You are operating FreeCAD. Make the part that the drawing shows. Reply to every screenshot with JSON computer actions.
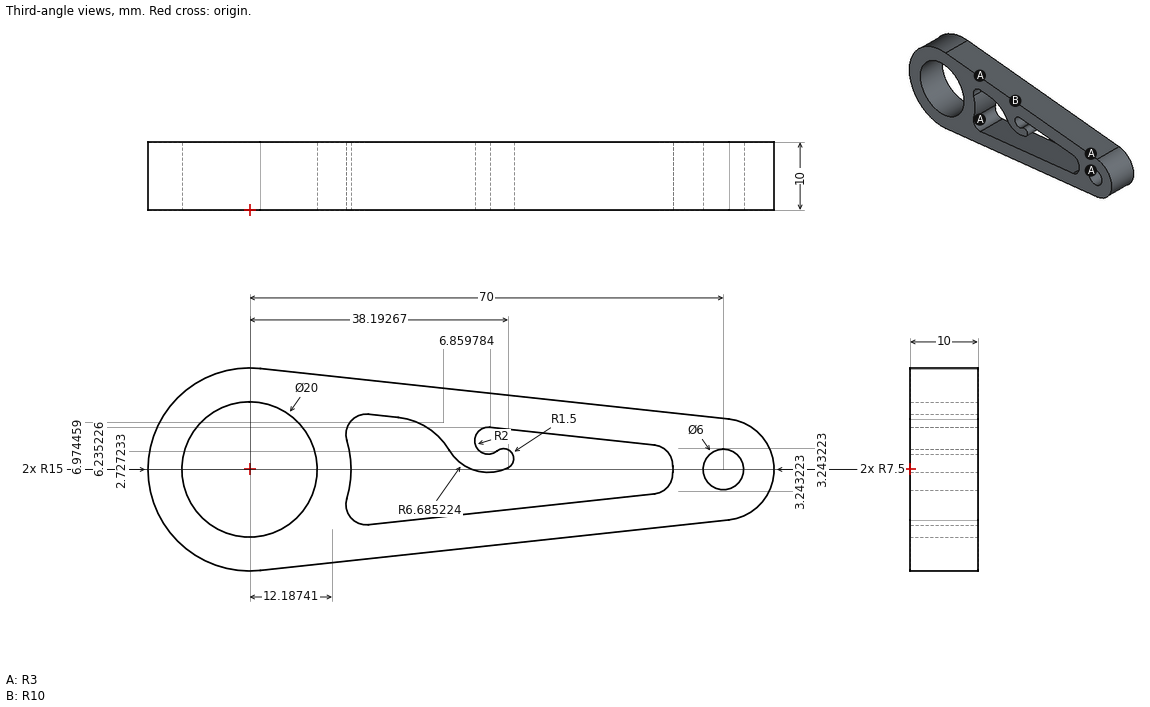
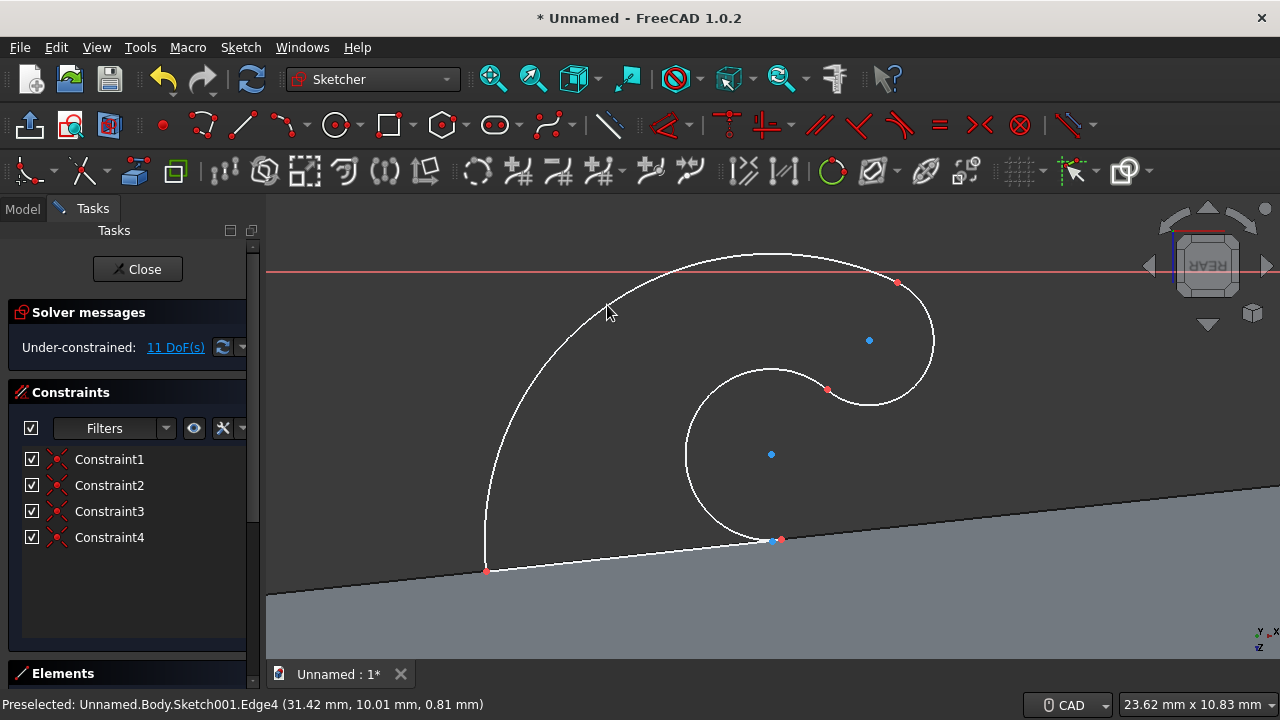
{"action": "left_click", "coordinate": [575, 562]}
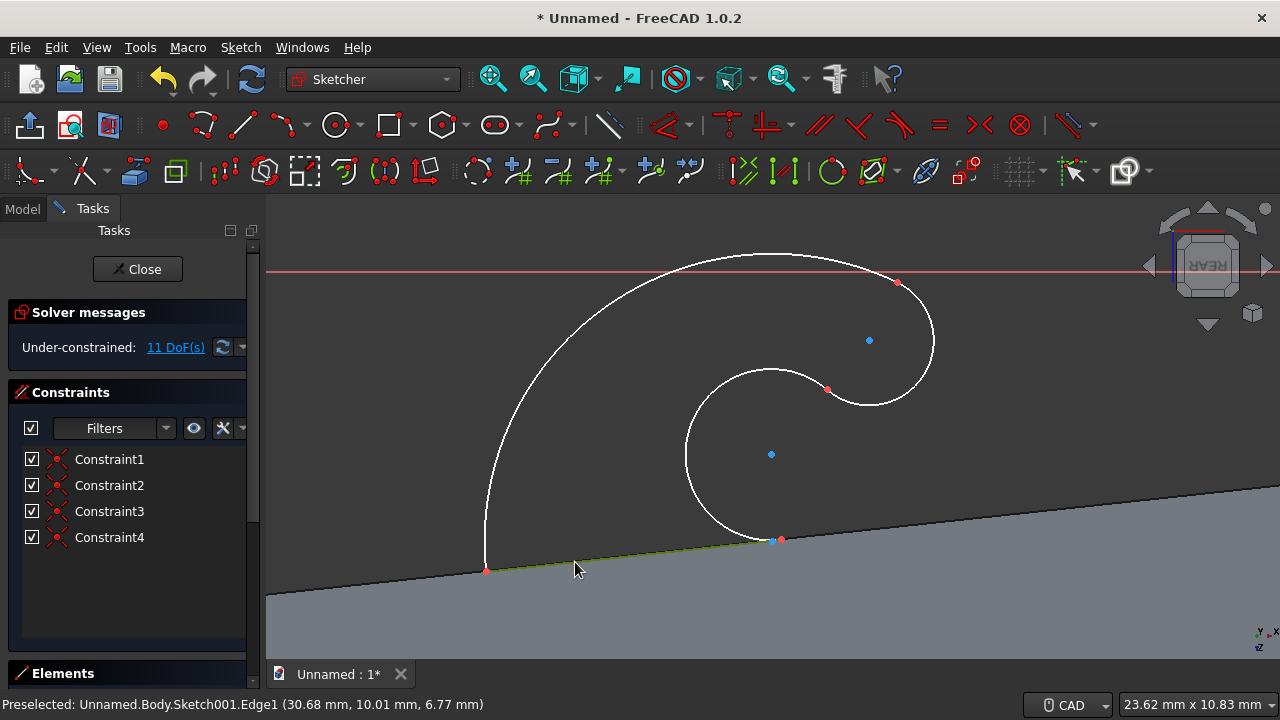
{"action": "left_click", "coordinate": [732, 379]}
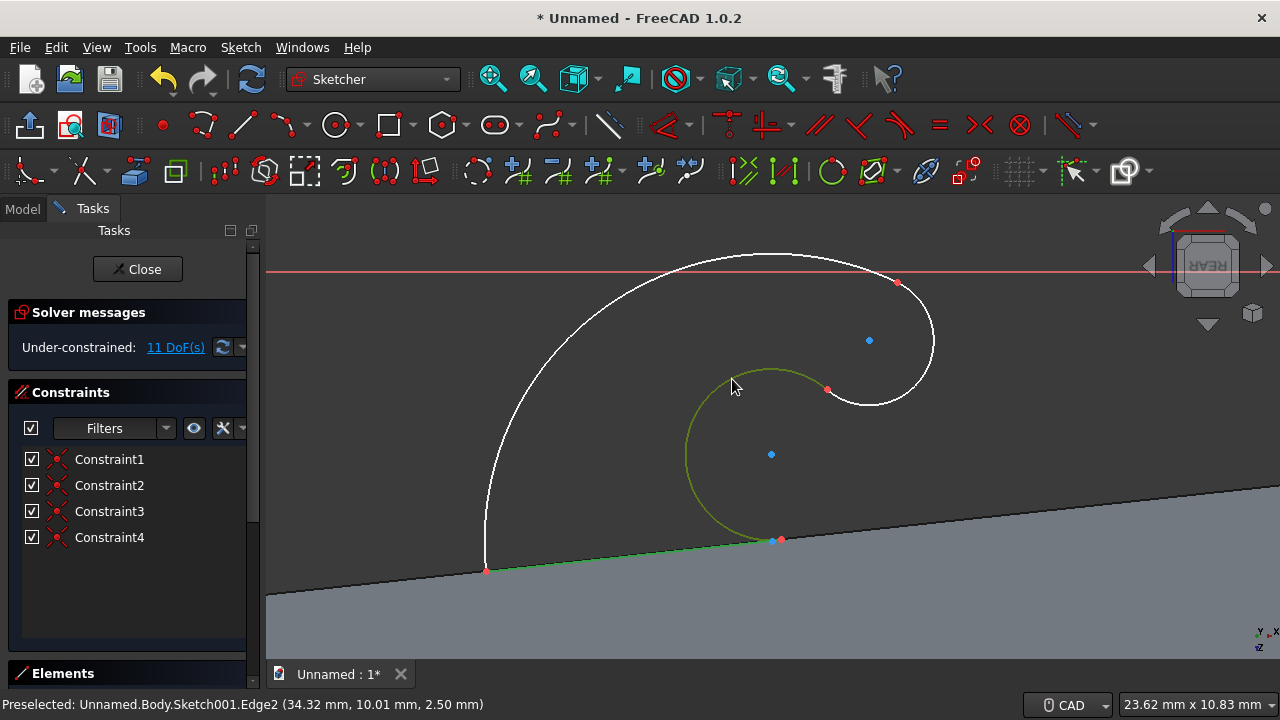
{"action": "left_click", "coordinate": [900, 126]}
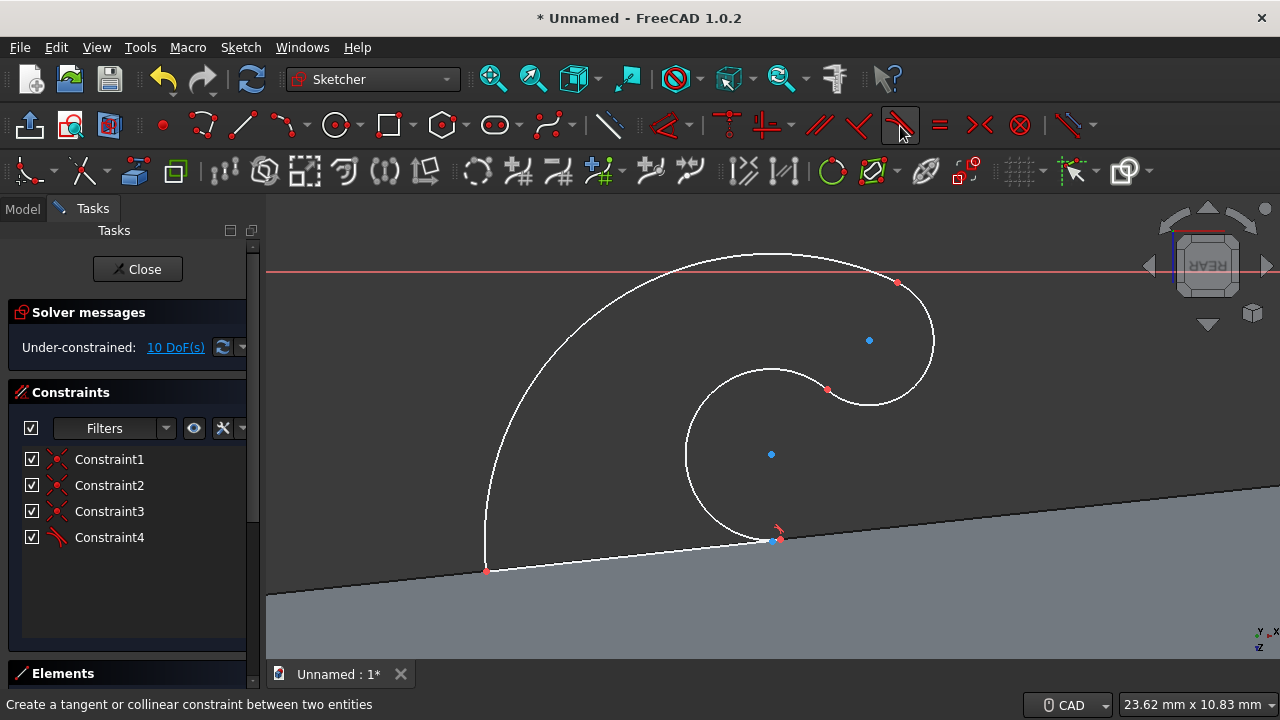
{"action": "left_click", "coordinate": [732, 379]}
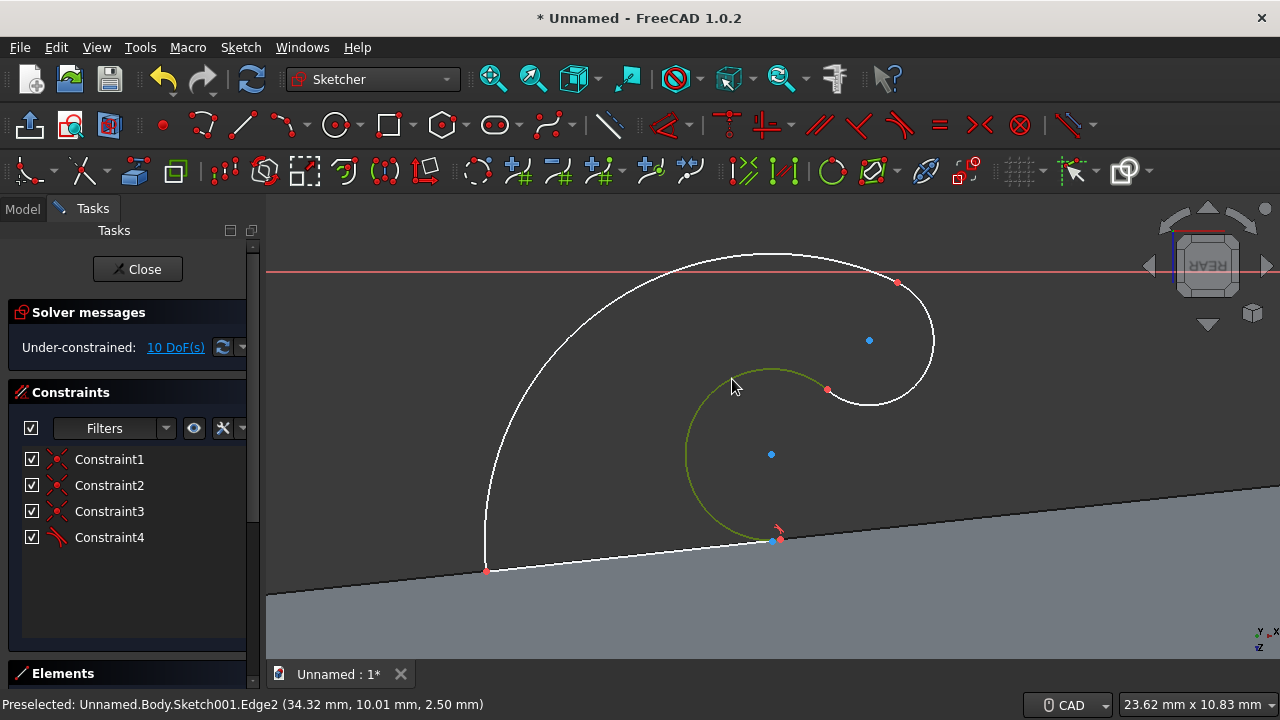
{"action": "left_click", "coordinate": [889, 402]}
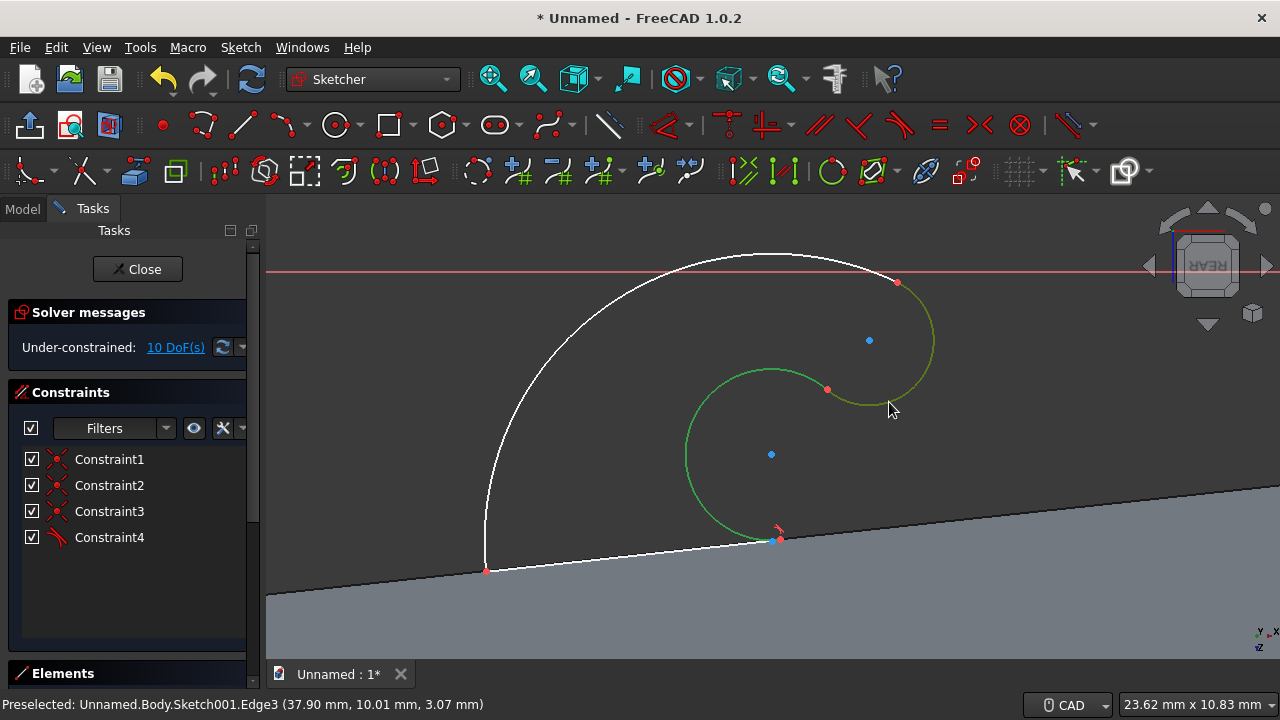
{"action": "left_click", "coordinate": [900, 126]}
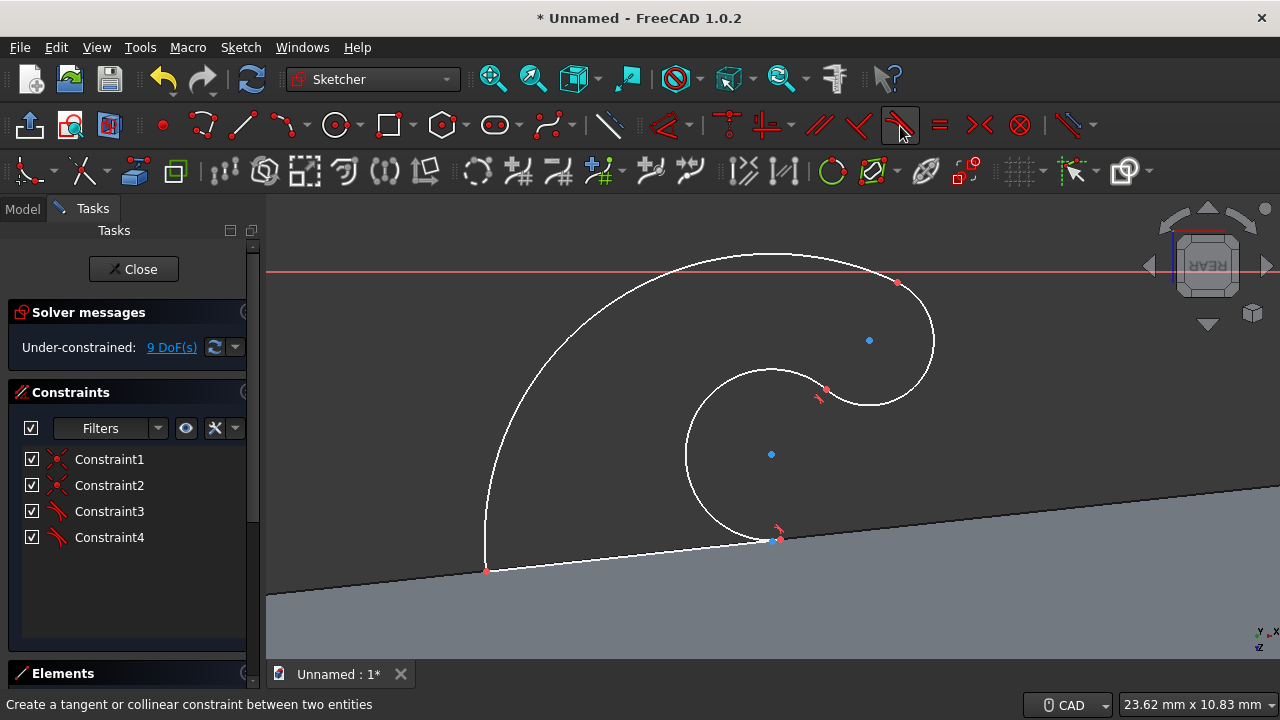
{"action": "left_click", "coordinate": [889, 402]}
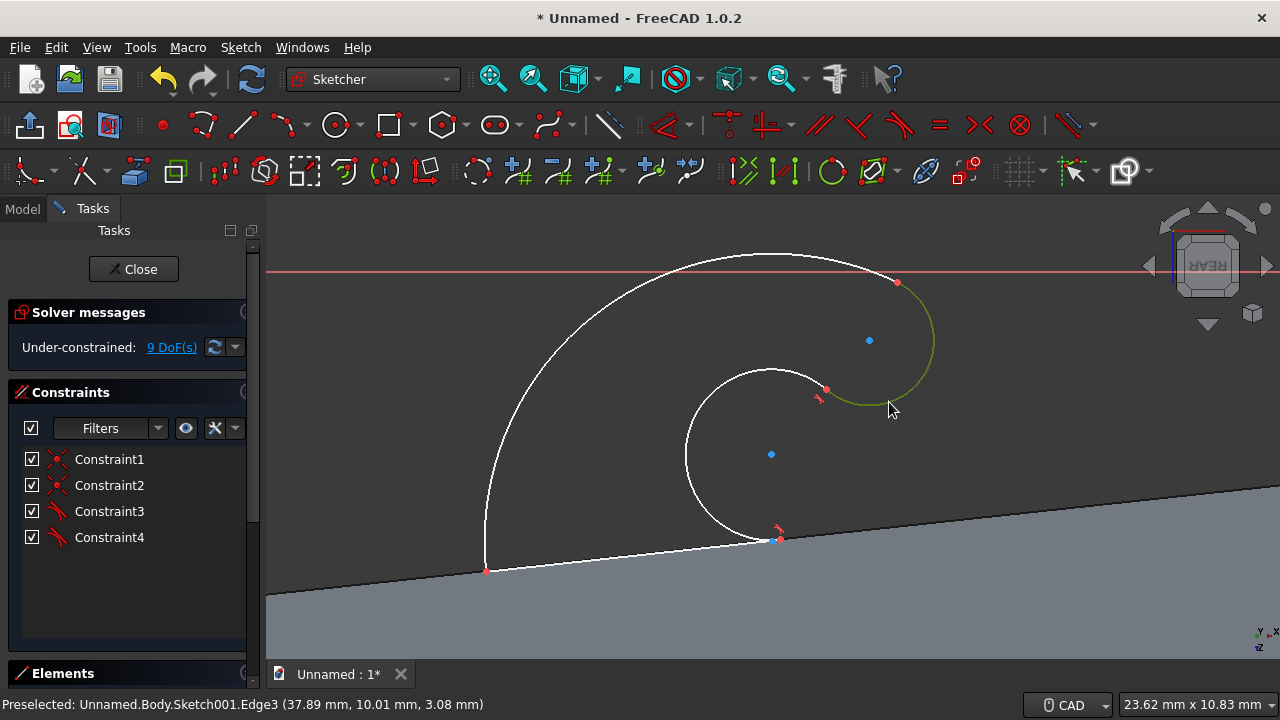
{"action": "left_click", "coordinate": [719, 259]}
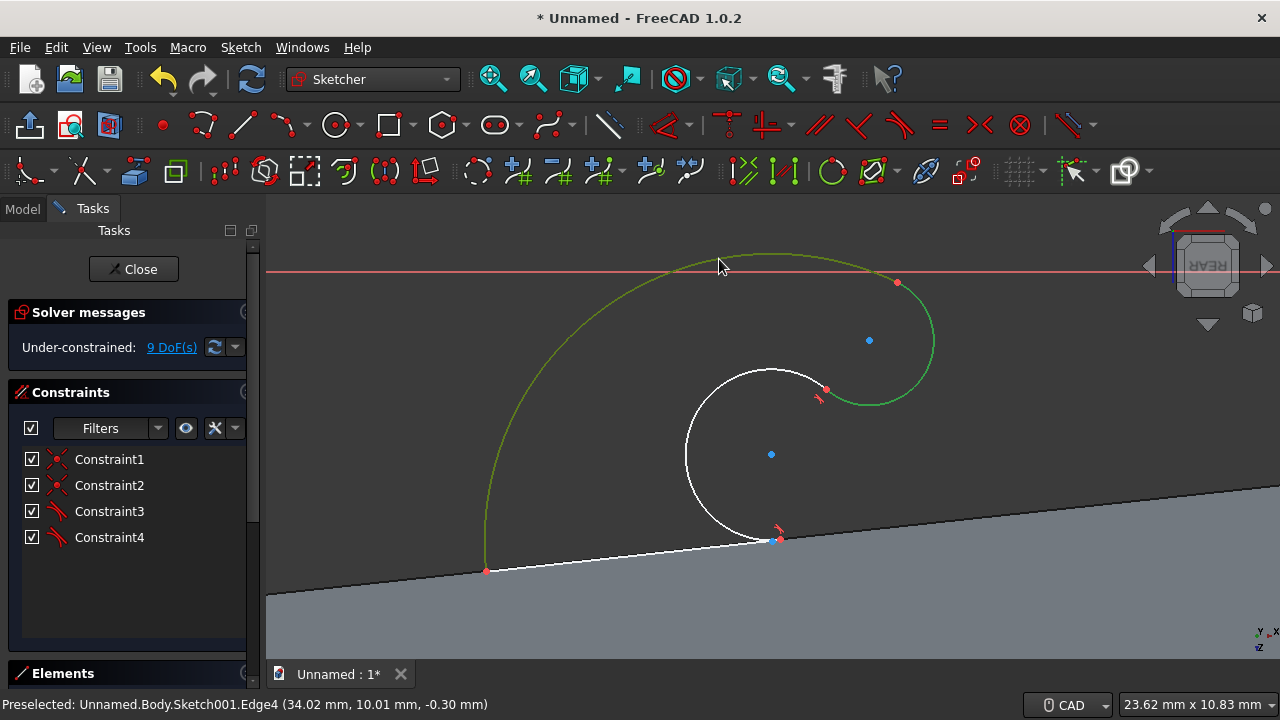
{"action": "left_click", "coordinate": [900, 126]}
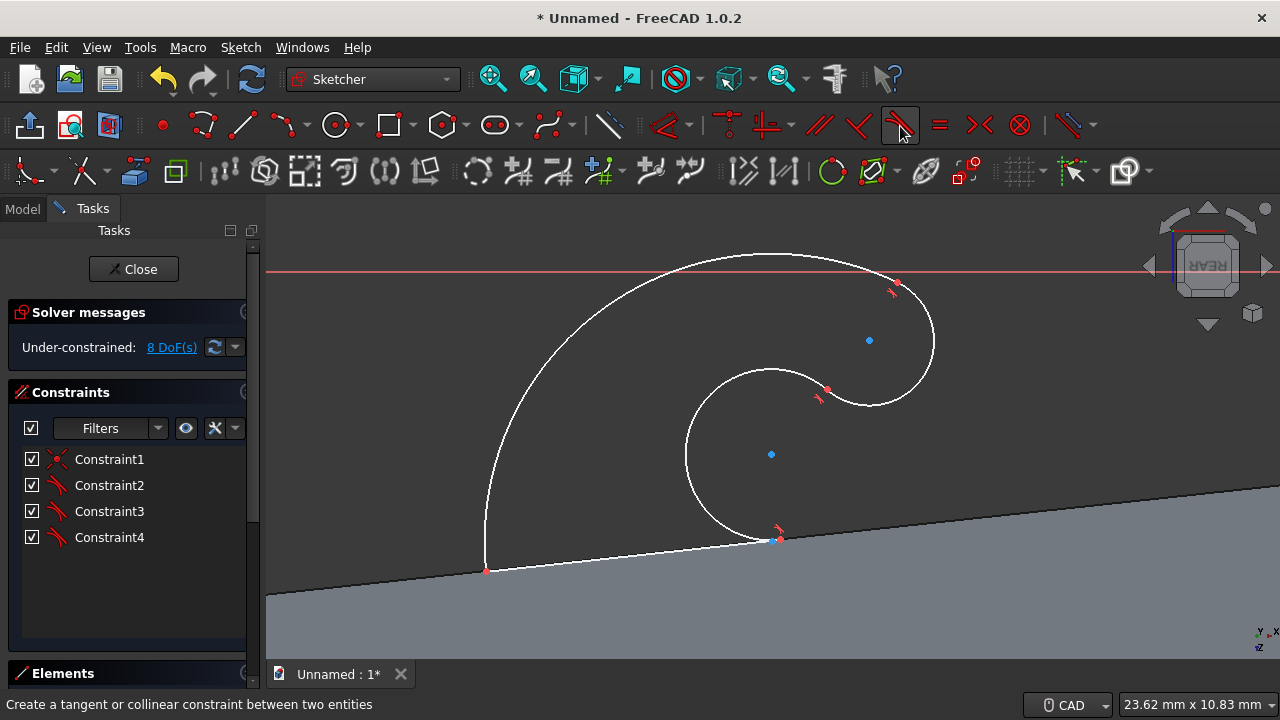
{"action": "left_click", "coordinate": [664, 126]}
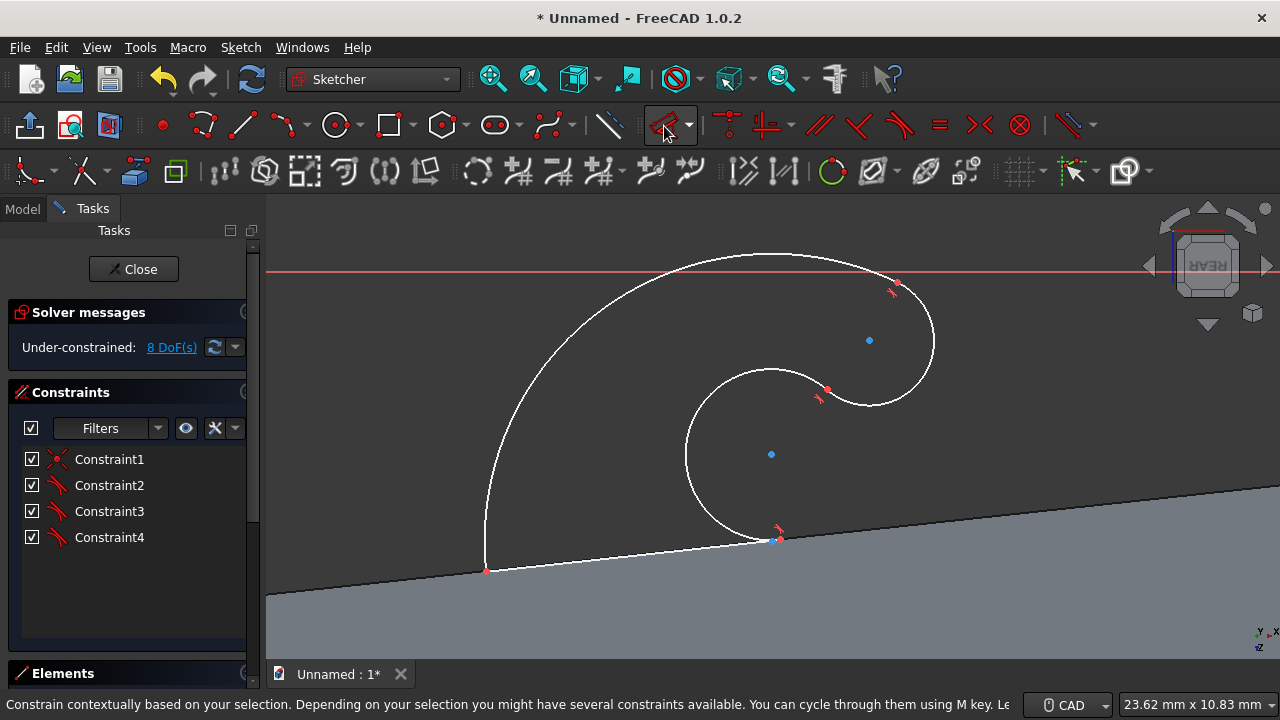
{"action": "left_click", "coordinate": [732, 379]}
{"action": "left_click", "coordinate": [717, 351]}